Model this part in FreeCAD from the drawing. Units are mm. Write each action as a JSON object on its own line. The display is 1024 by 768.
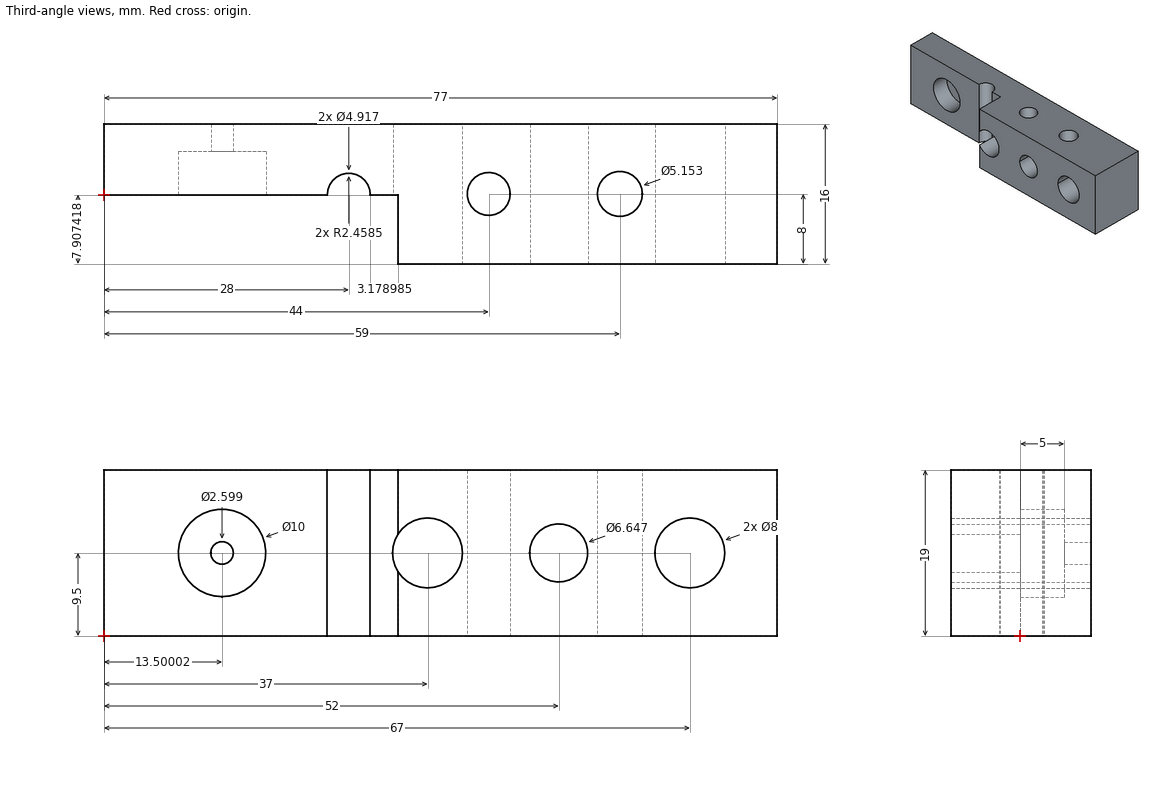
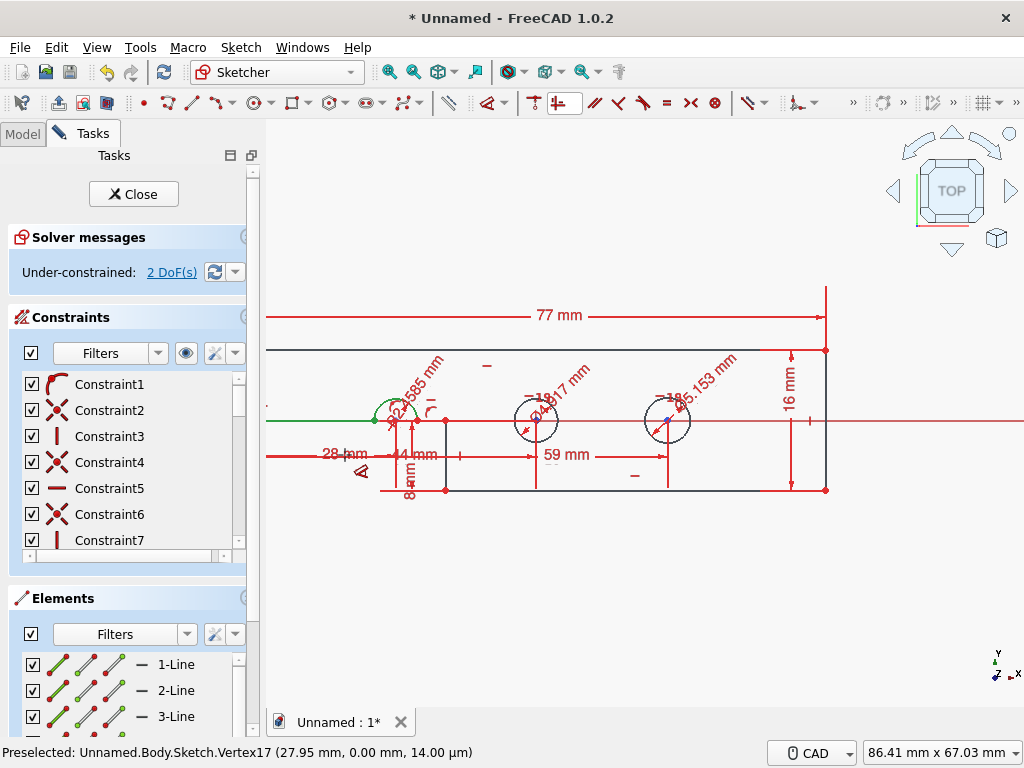
{"action": "scroll", "coordinate": [429, 421], "scroll_direction": "up", "scroll_amount": 2}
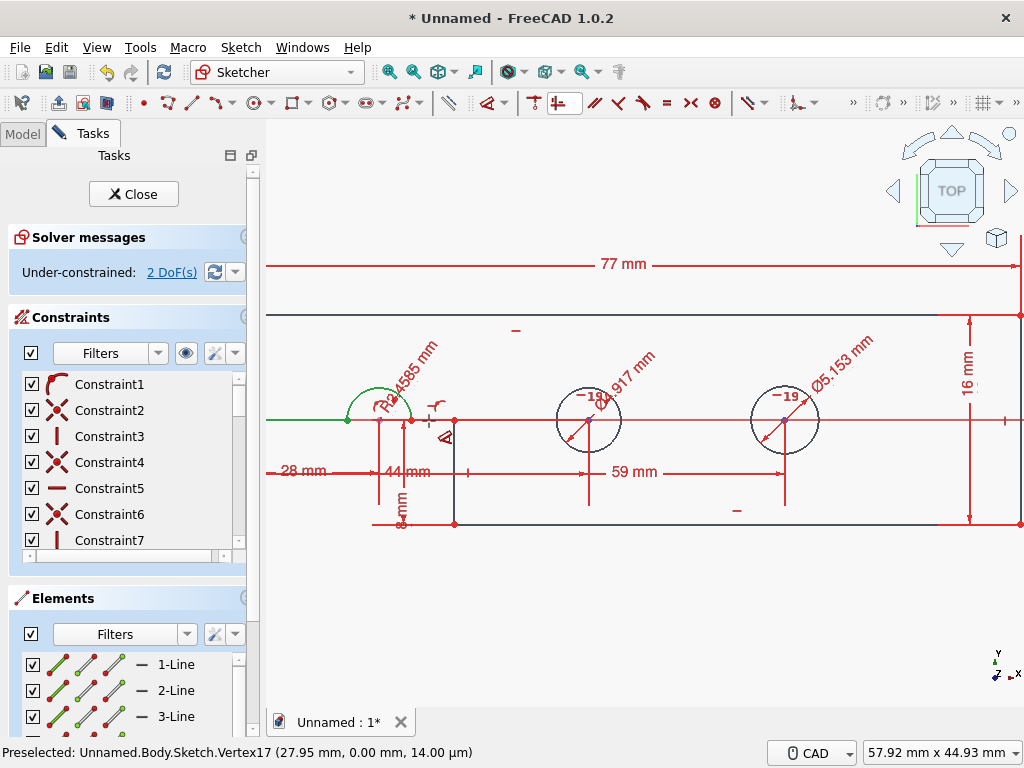
{"action": "left_click", "coordinate": [429, 420]}
{"action": "left_click", "coordinate": [433, 338]}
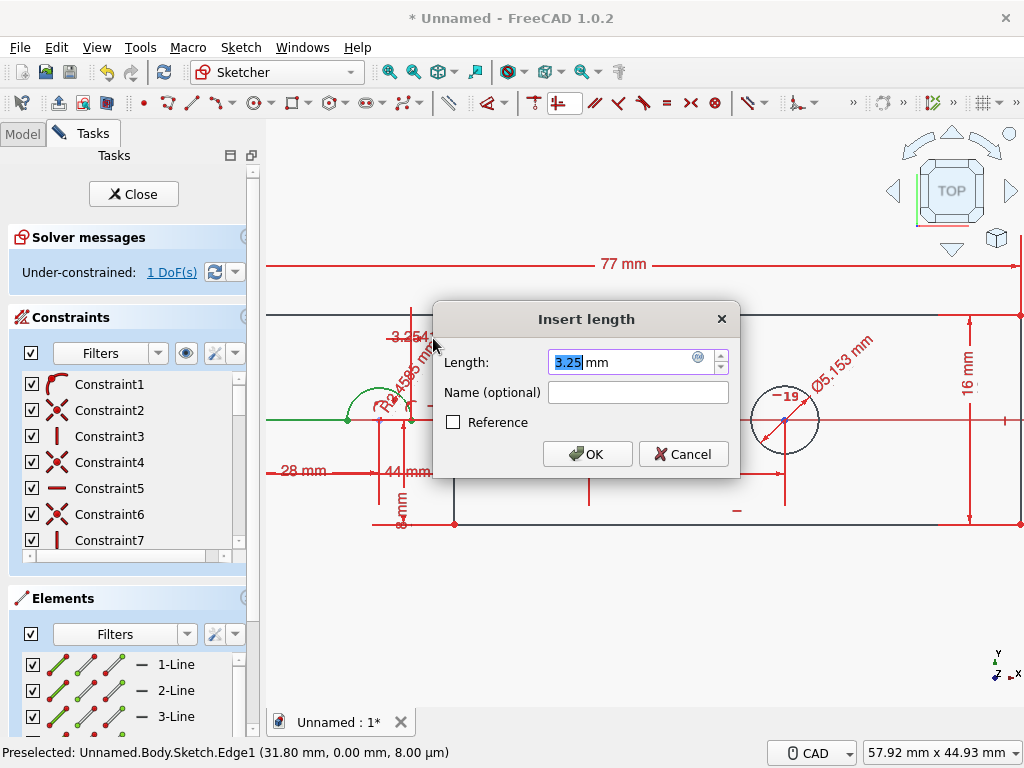
{"action": "type", "text": "3.178985"}
{"action": "key", "text": "Return"}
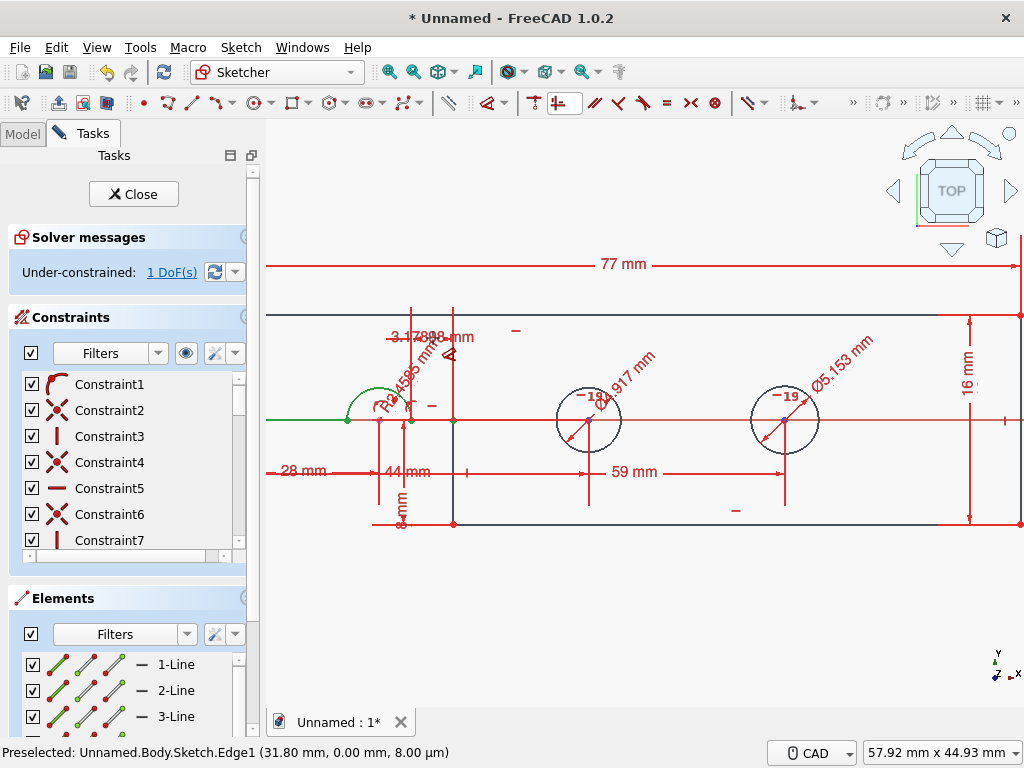
{"action": "left_click", "coordinate": [453, 452]}
{"action": "left_click", "coordinate": [419, 448]}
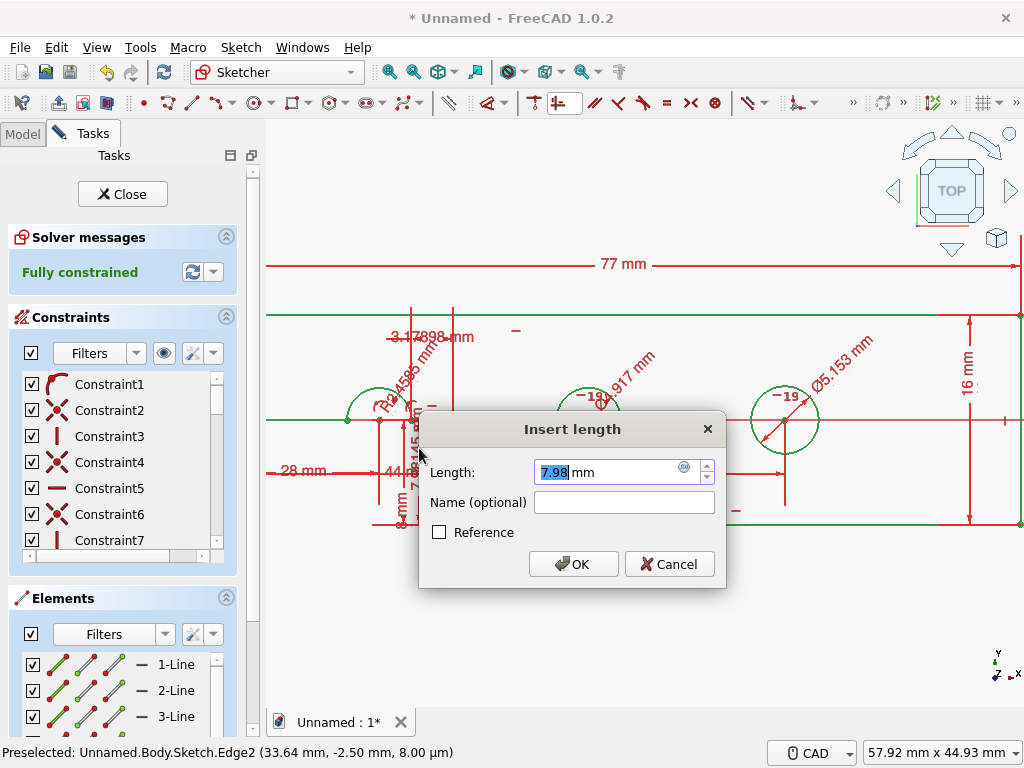
{"action": "type", "text": "7.907418"}
{"action": "key", "text": "Return"}
{"action": "key", "text": "Escape"}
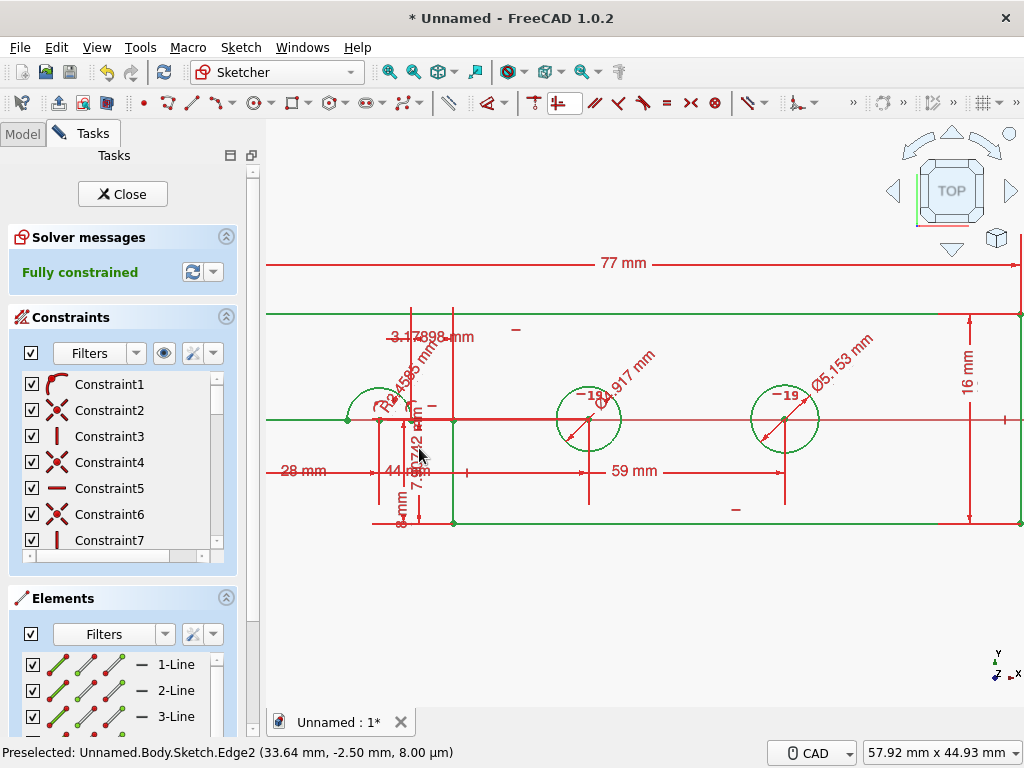
{"action": "left_click", "coordinate": [123, 194]}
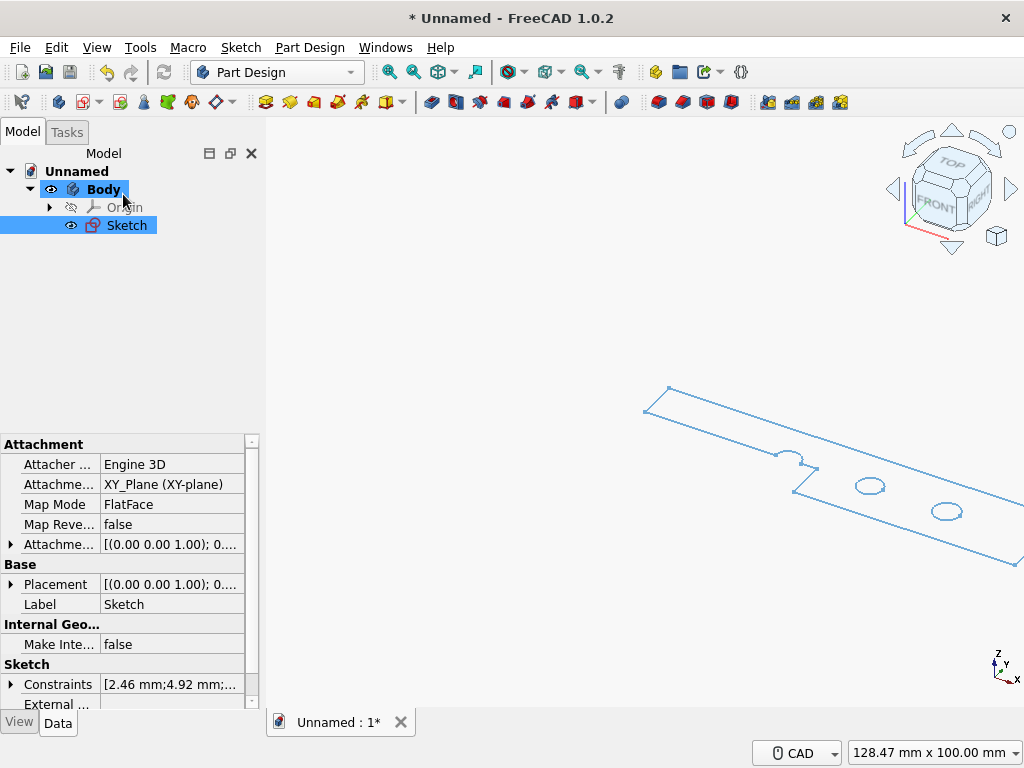
{"action": "left_click", "coordinate": [266, 102]}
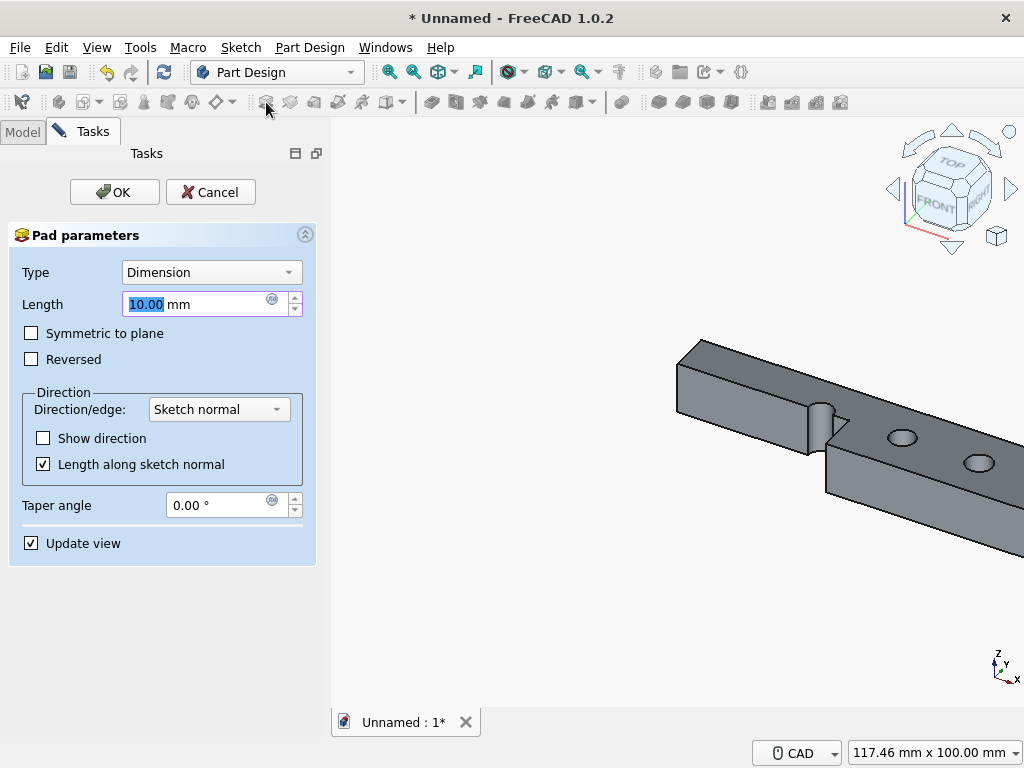
{"action": "type", "text": "19"}
{"action": "key", "text": "Tab"}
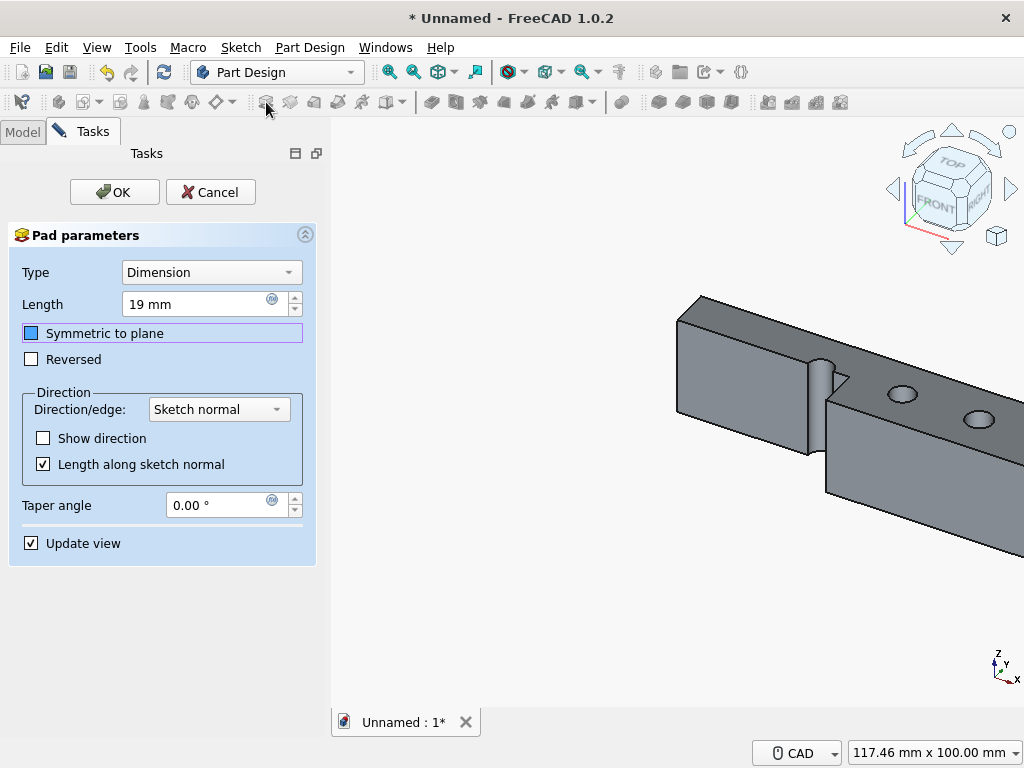
{"action": "left_click", "coordinate": [115, 192]}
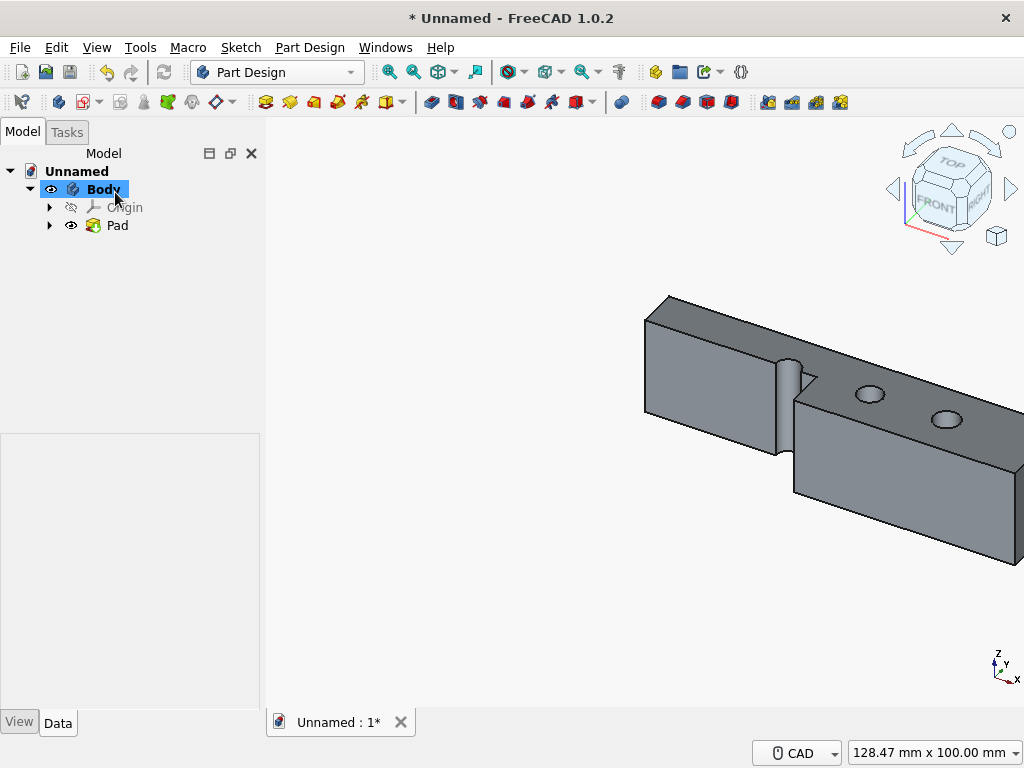
{"action": "left_click", "coordinate": [390, 72]}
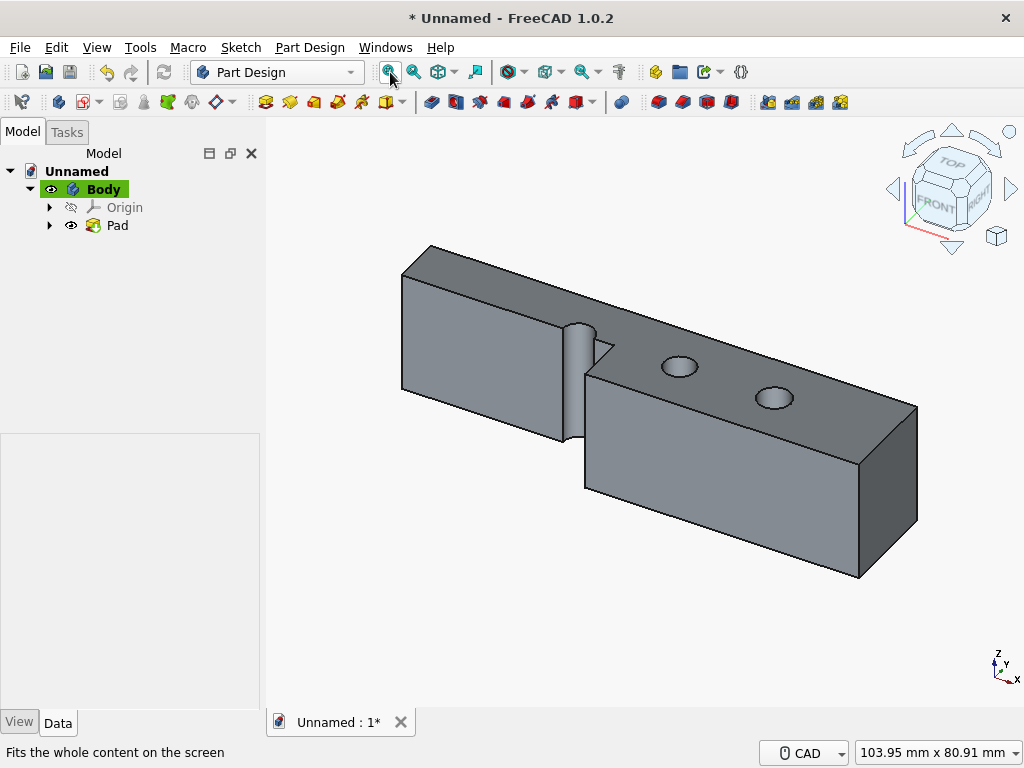
{"action": "key", "text": "4"}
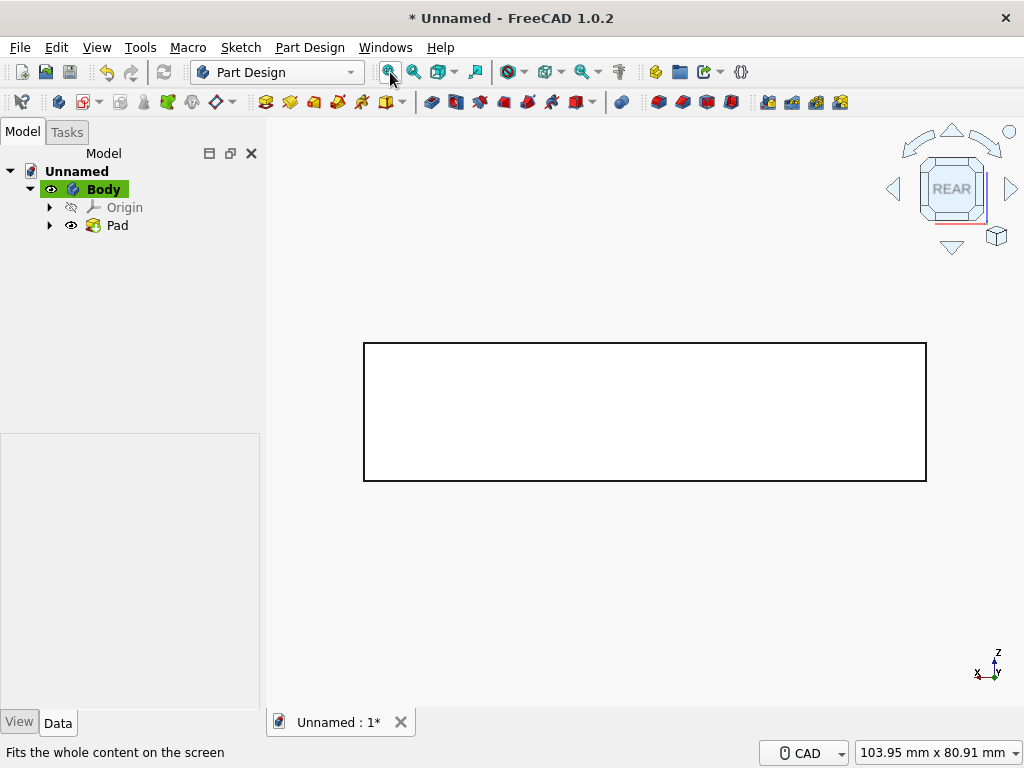
{"action": "left_click", "coordinate": [485, 411]}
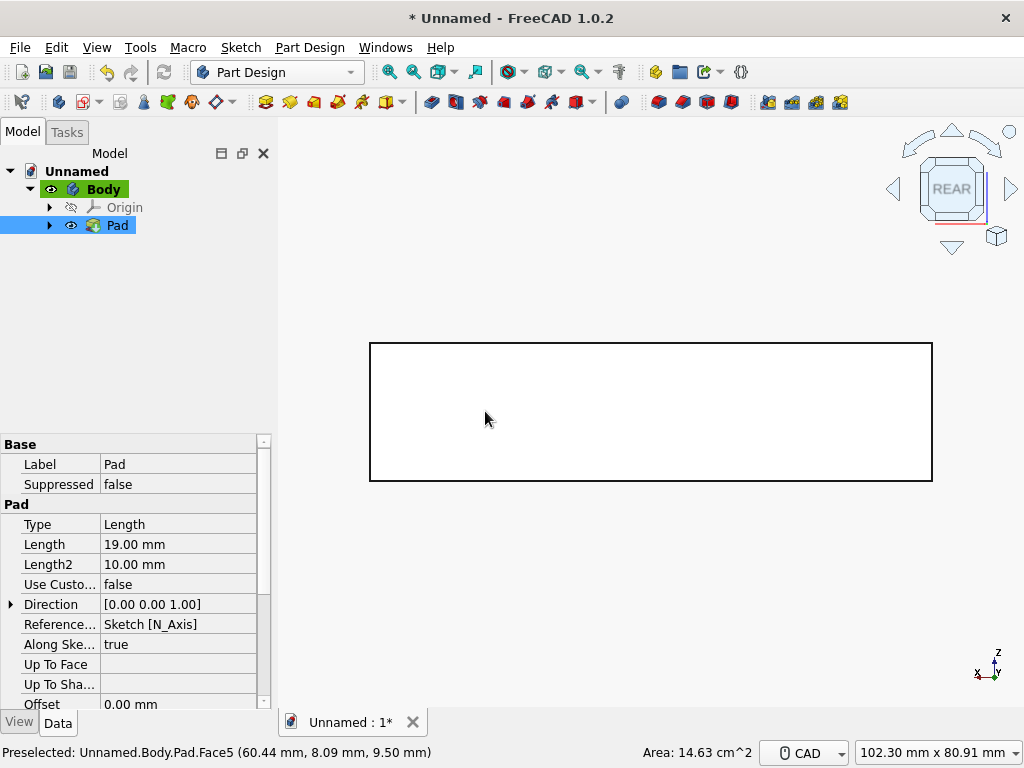
{"action": "left_click", "coordinate": [84, 102]}